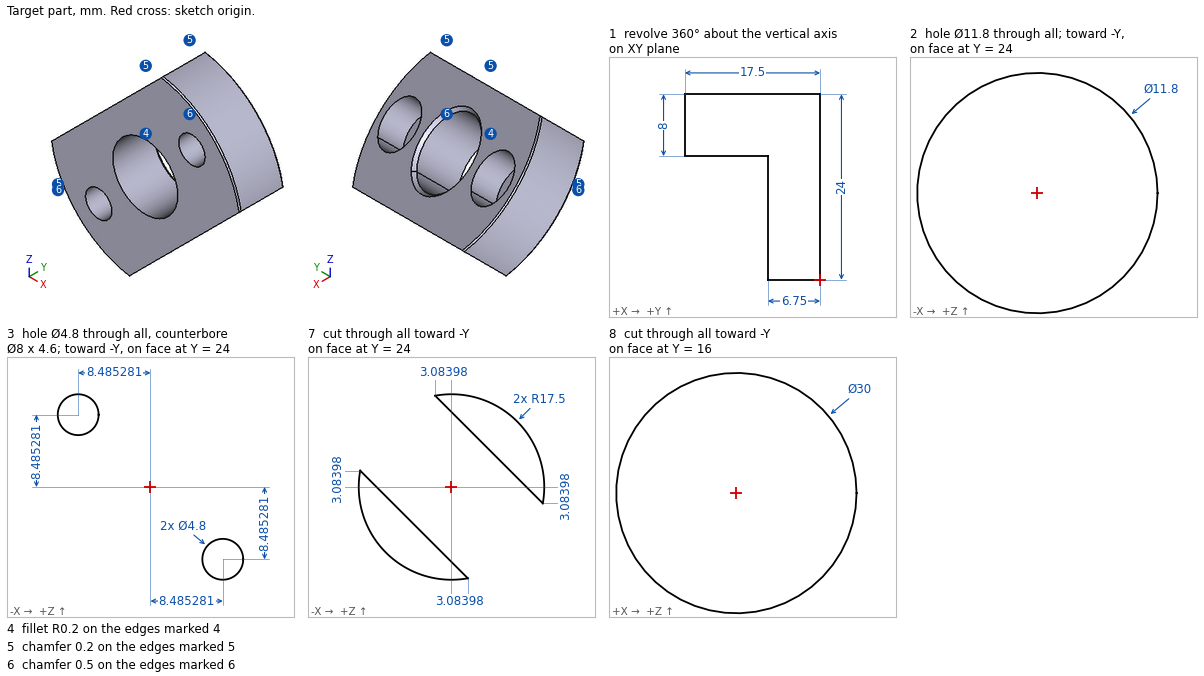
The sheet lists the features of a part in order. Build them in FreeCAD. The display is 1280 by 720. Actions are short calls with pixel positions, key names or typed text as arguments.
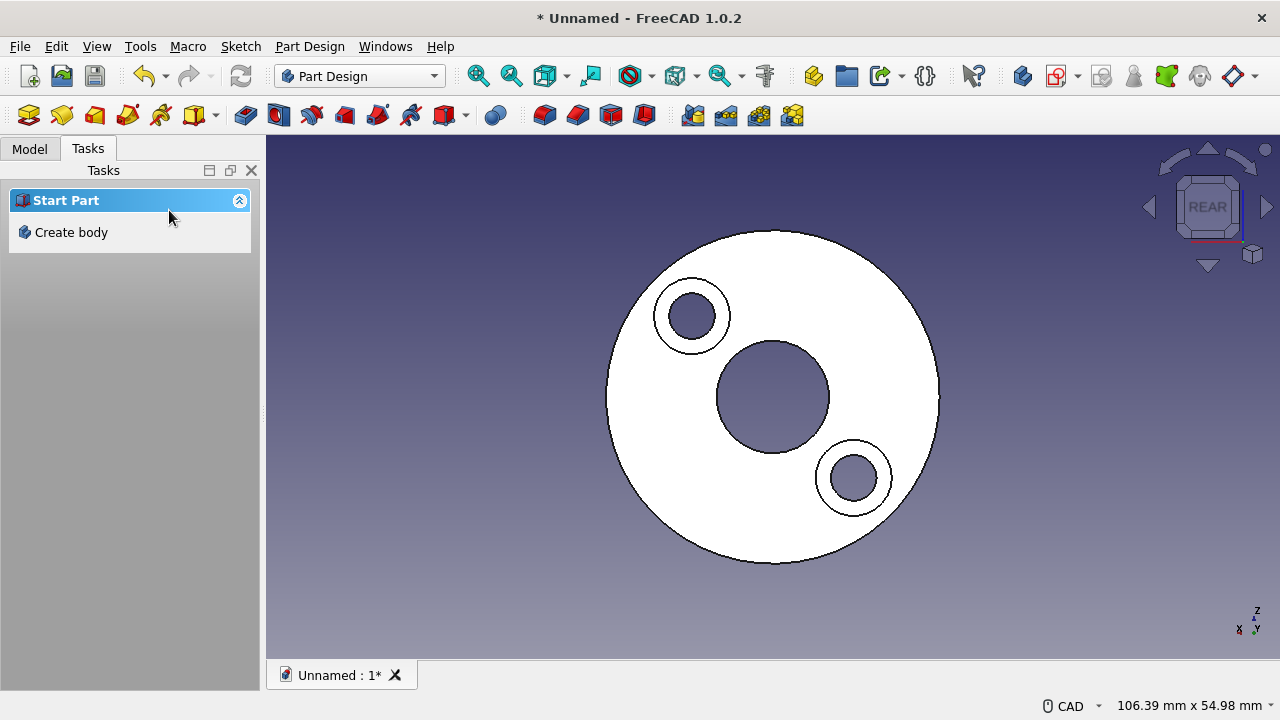
key(0)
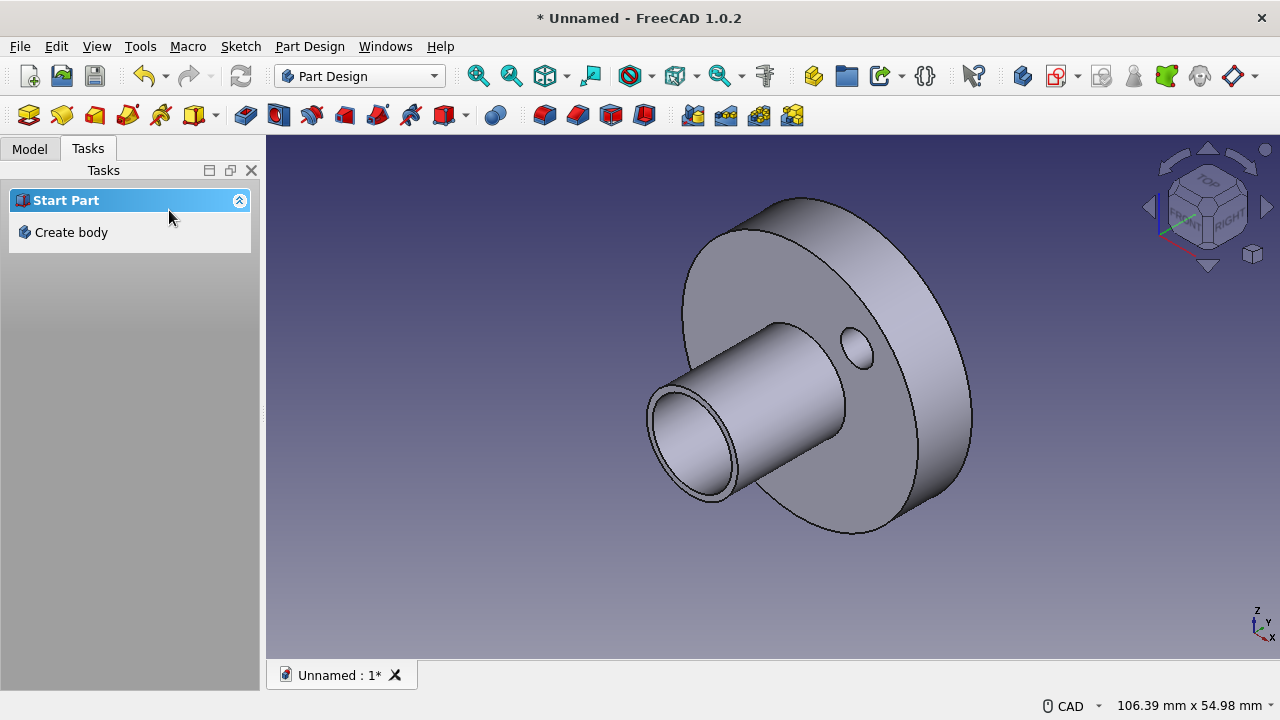
key(2)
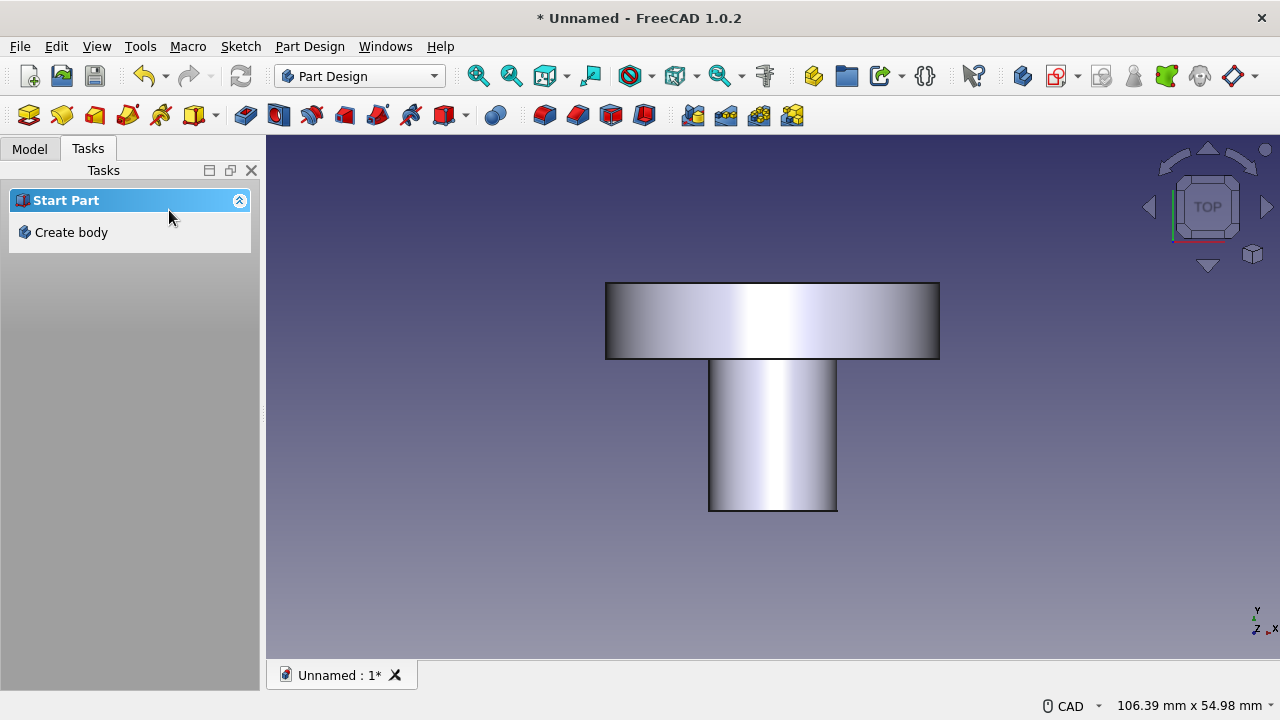
click(479, 76)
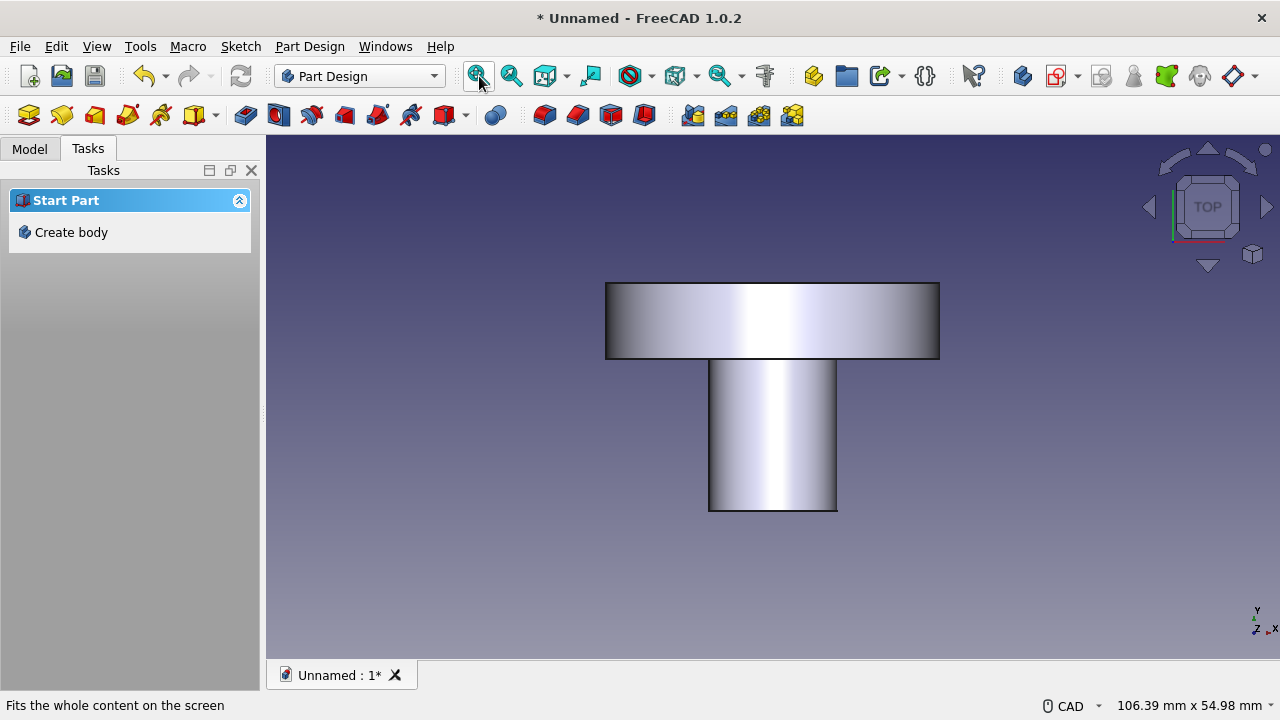
key(1)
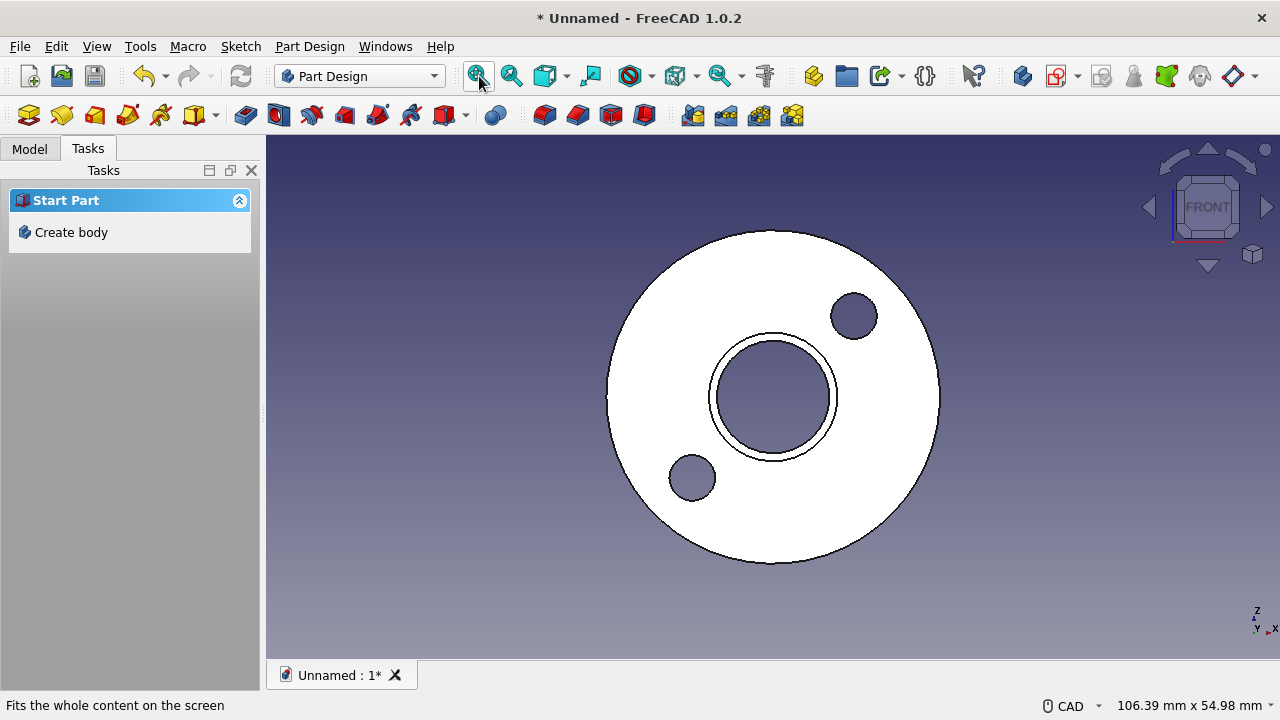
key(3)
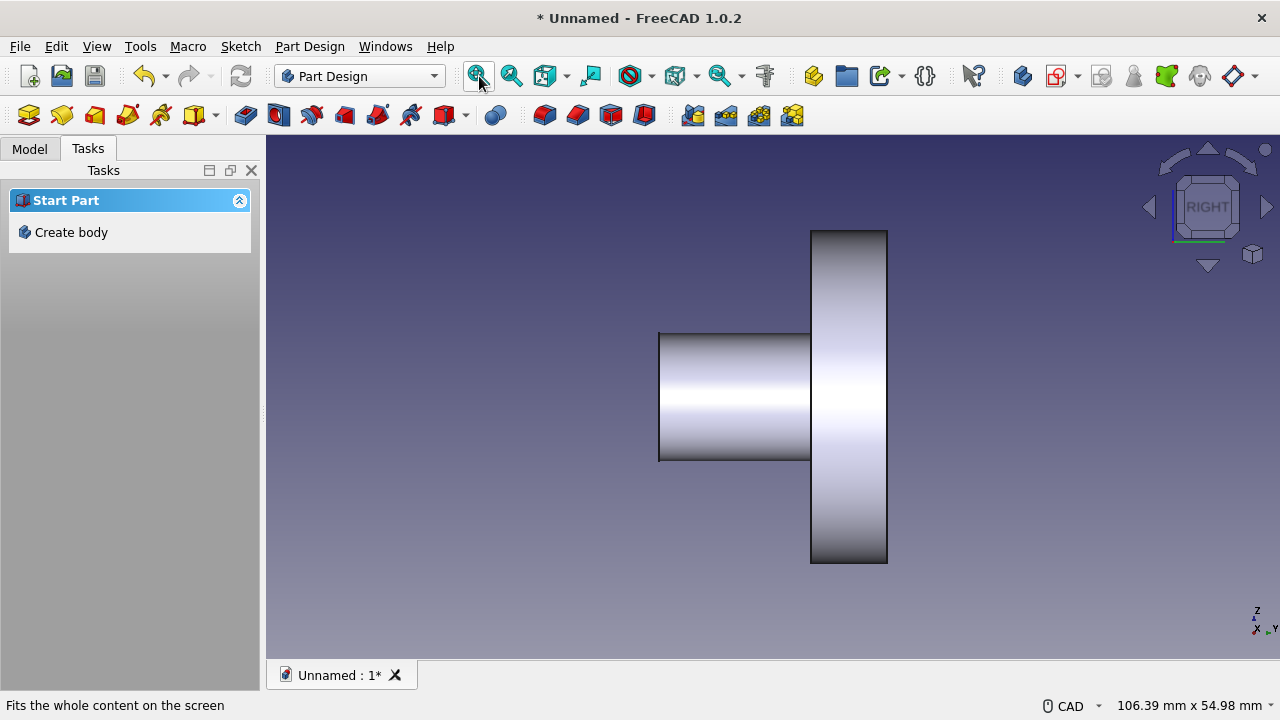
key(5)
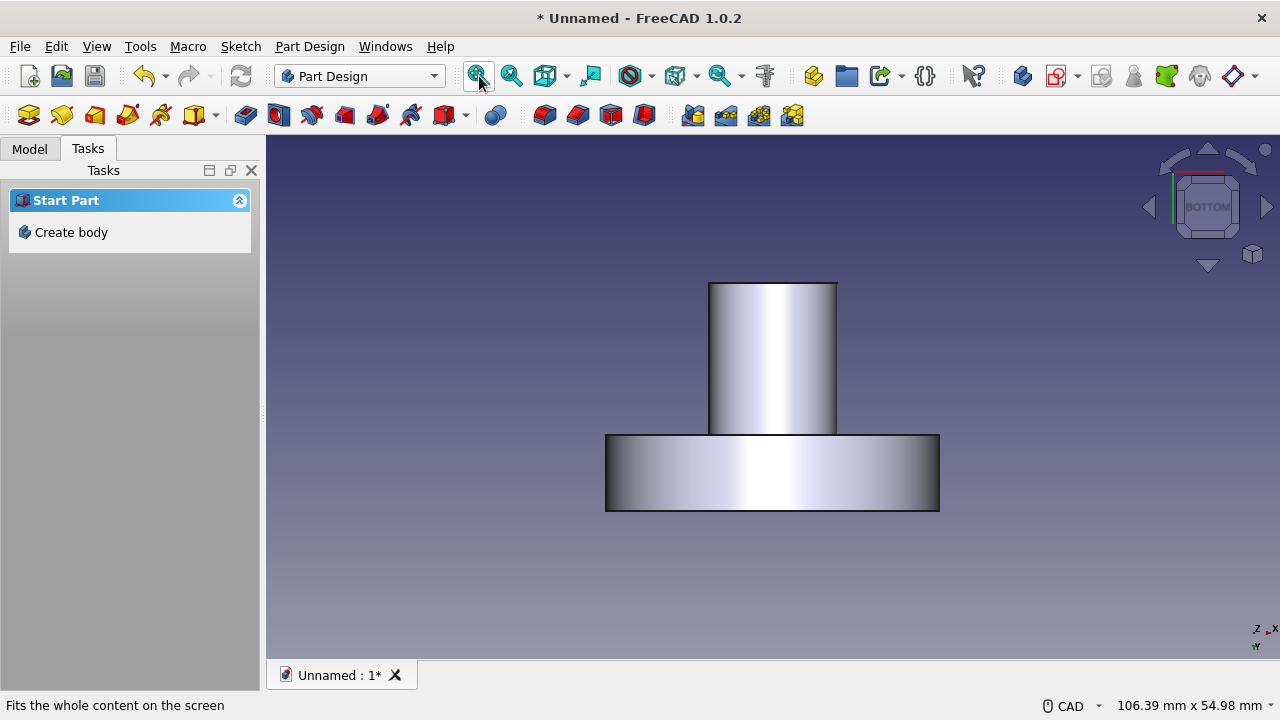
click(479, 76)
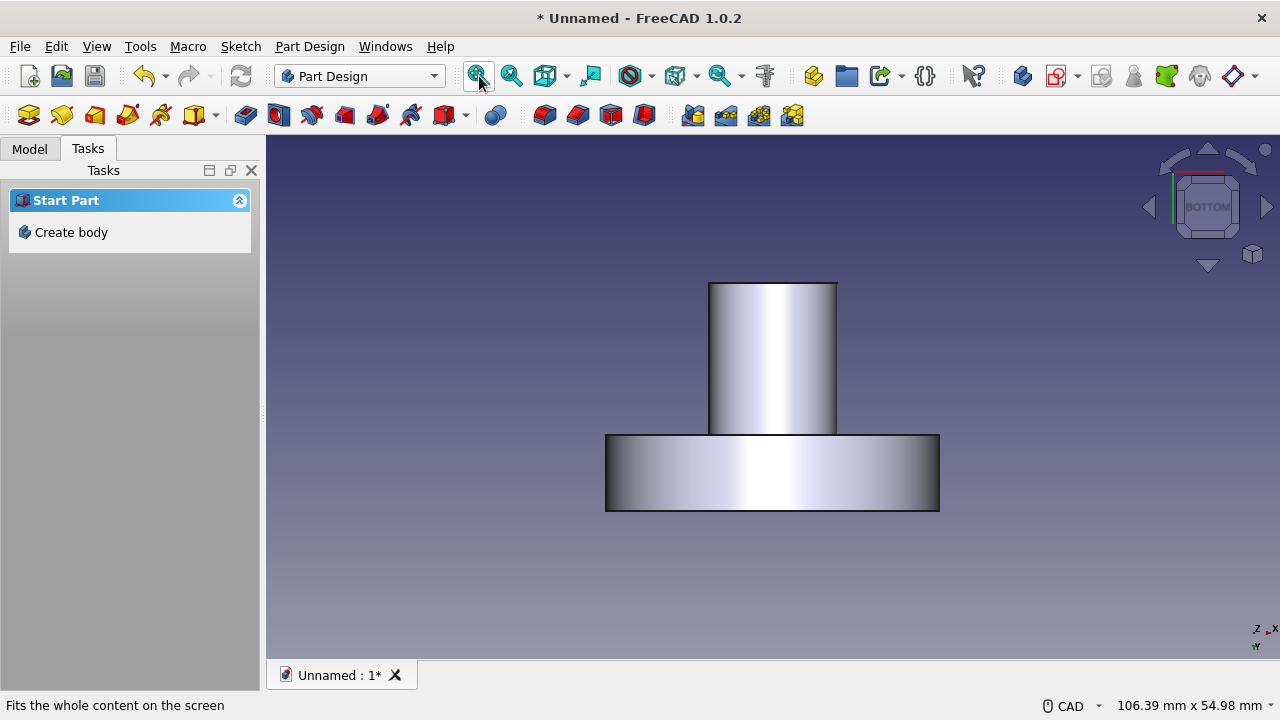
key(4)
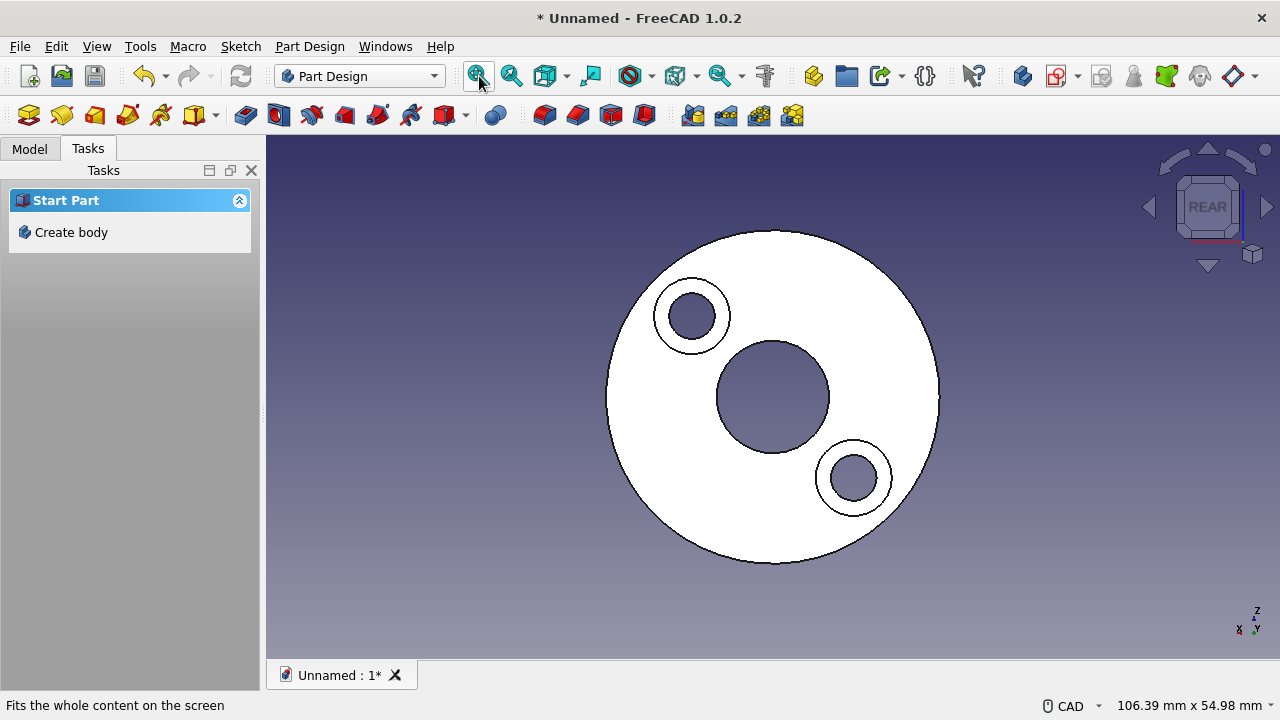
key(6)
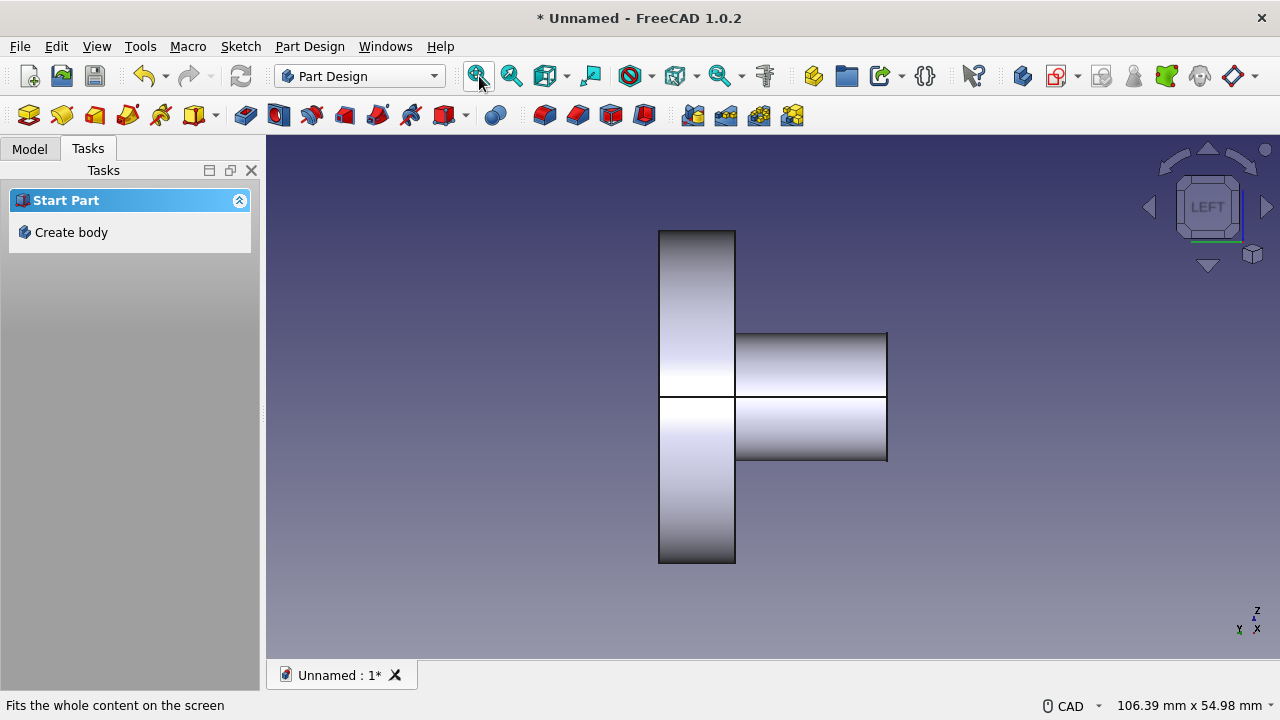
key(v)
key(3)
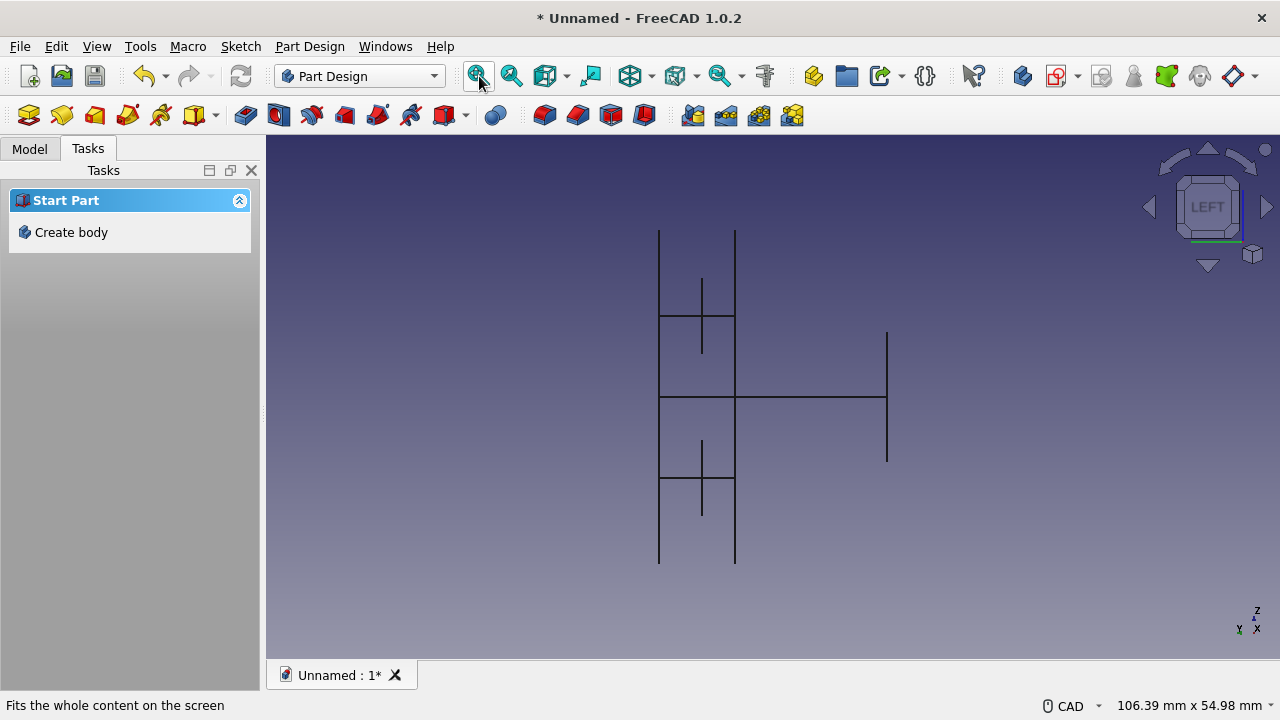
key(0)